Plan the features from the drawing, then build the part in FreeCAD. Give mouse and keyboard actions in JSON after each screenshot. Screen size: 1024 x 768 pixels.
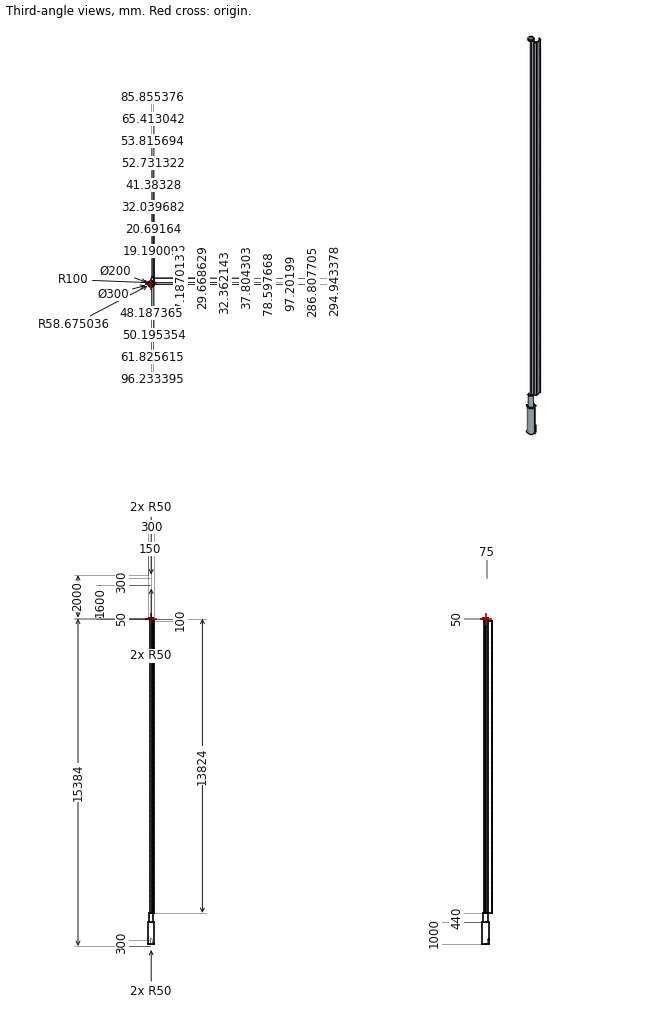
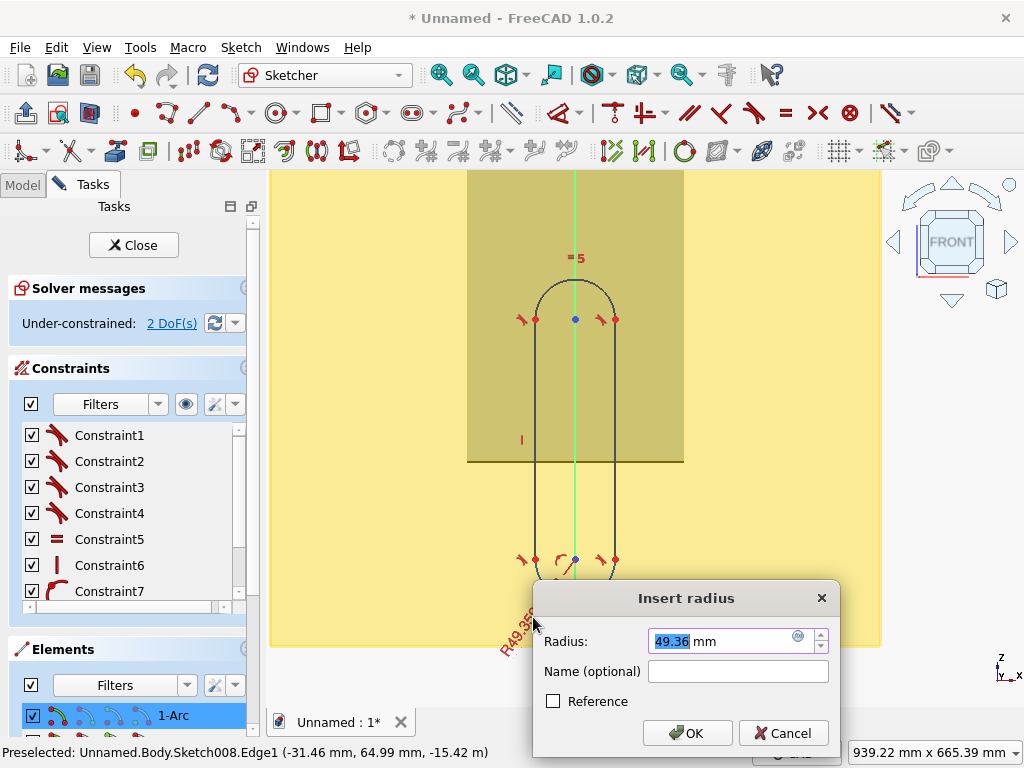
{"action": "type", "text": "50"}
{"action": "key", "text": "Return"}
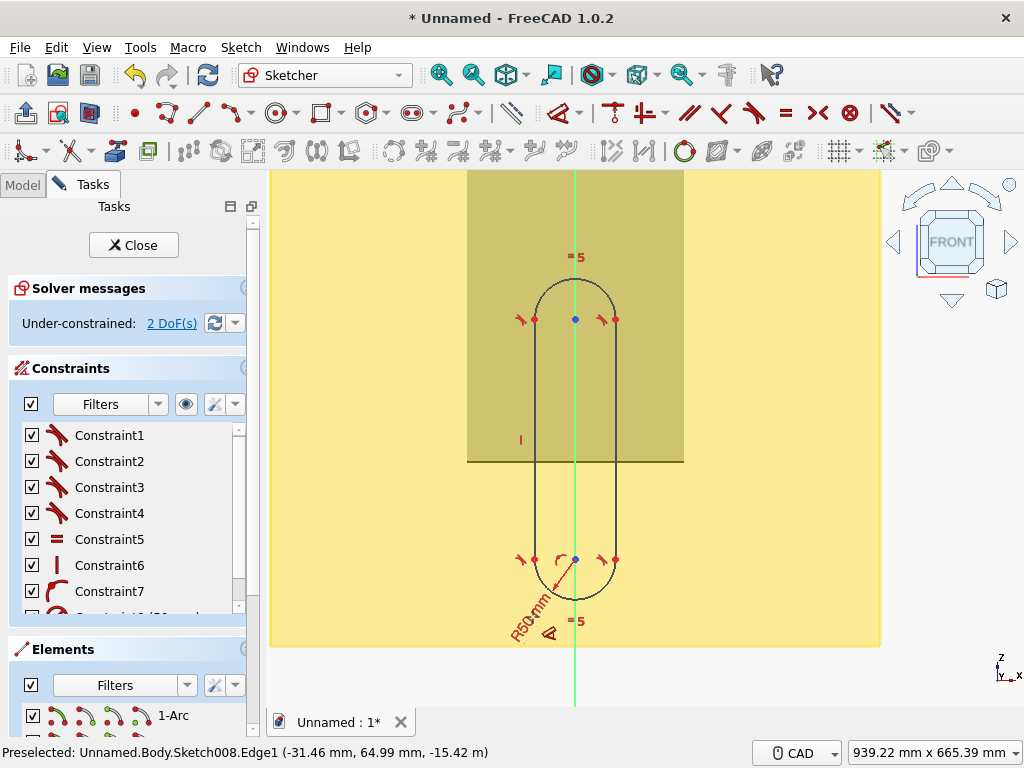
{"action": "left_click", "coordinate": [535, 487]}
{"action": "left_click", "coordinate": [501, 439]}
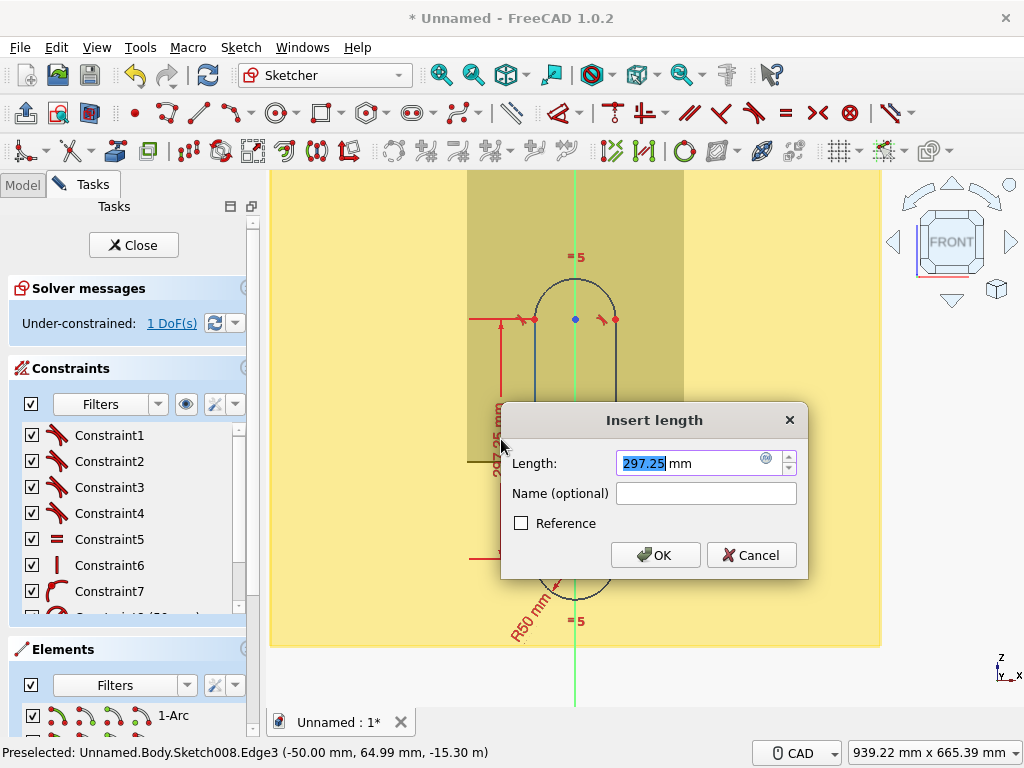
{"action": "type", "text": "300"}
{"action": "key", "text": "Return"}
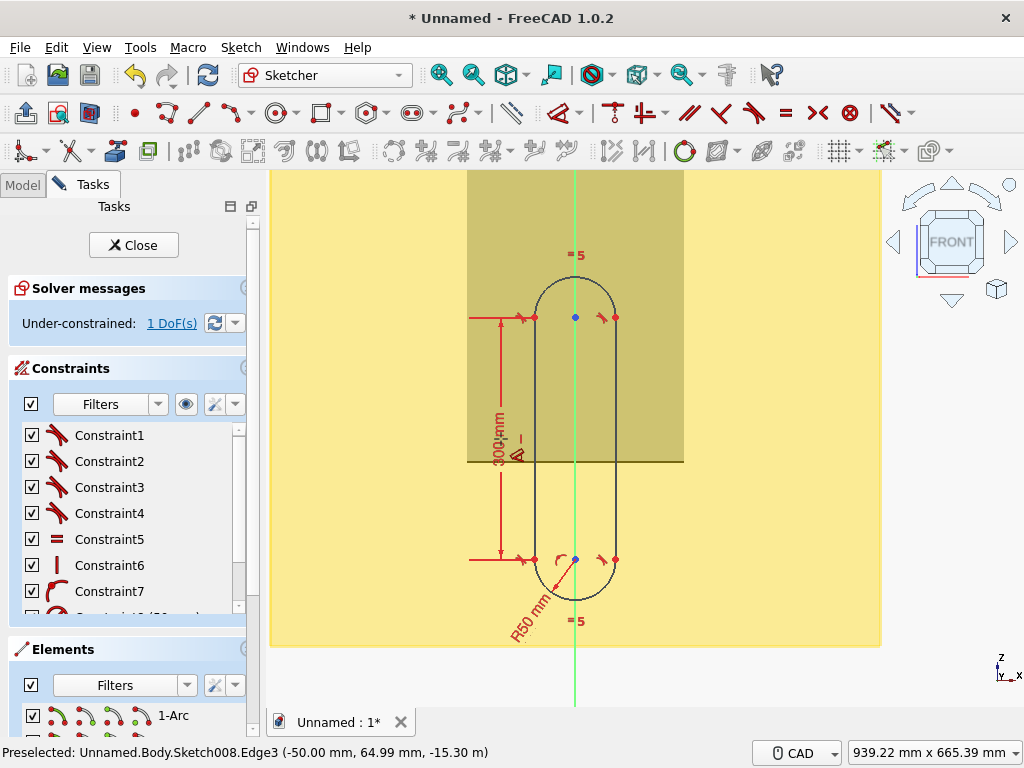
{"action": "left_click", "coordinate": [535, 560]}
{"action": "left_click", "coordinate": [501, 379]}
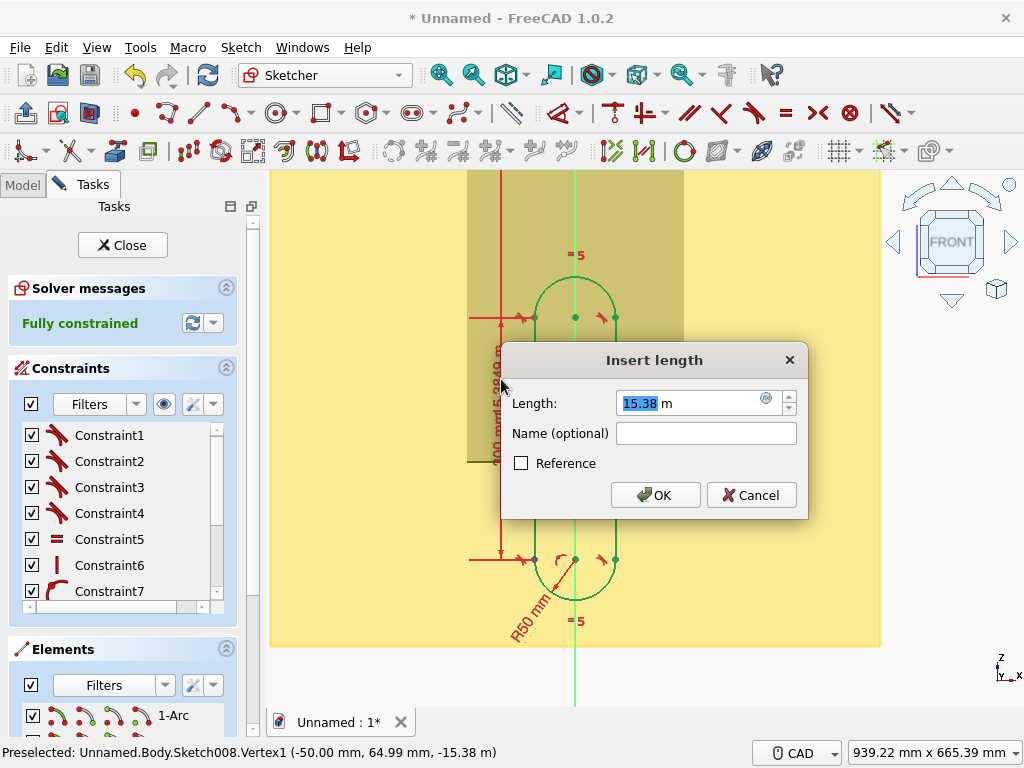
{"action": "key", "text": "ctrl+a"}
{"action": "type", "text": "15384 mm"}
{"action": "key", "text": "Return"}
{"action": "key", "text": "Escape"}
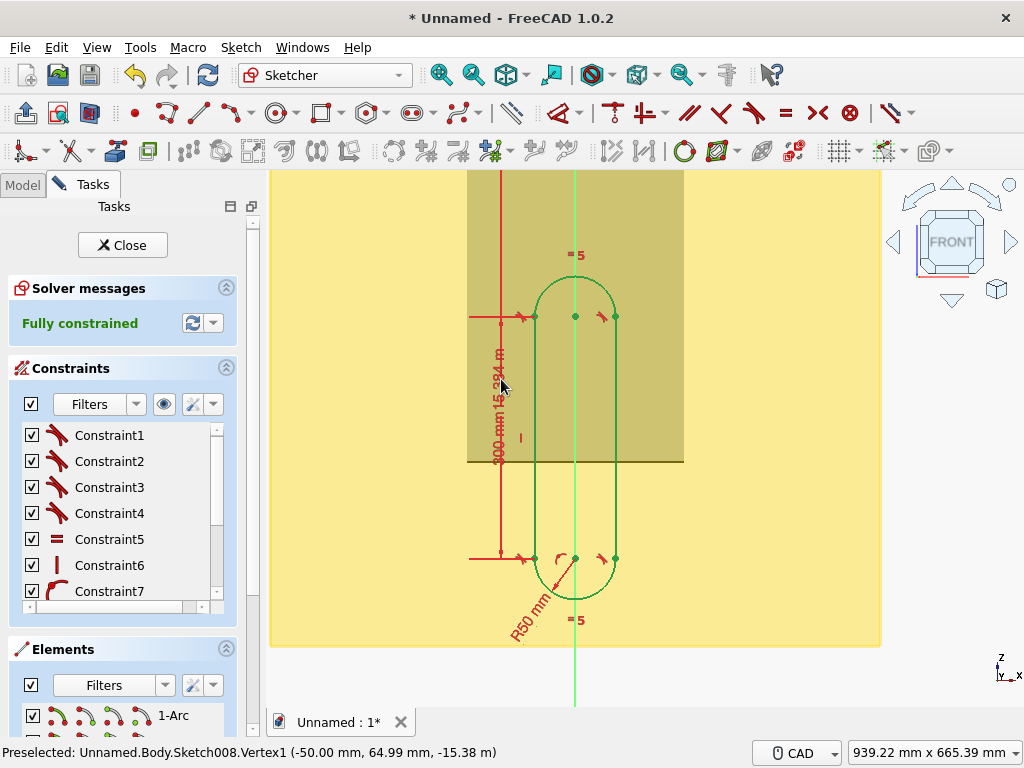
{"action": "left_click", "coordinate": [123, 245]}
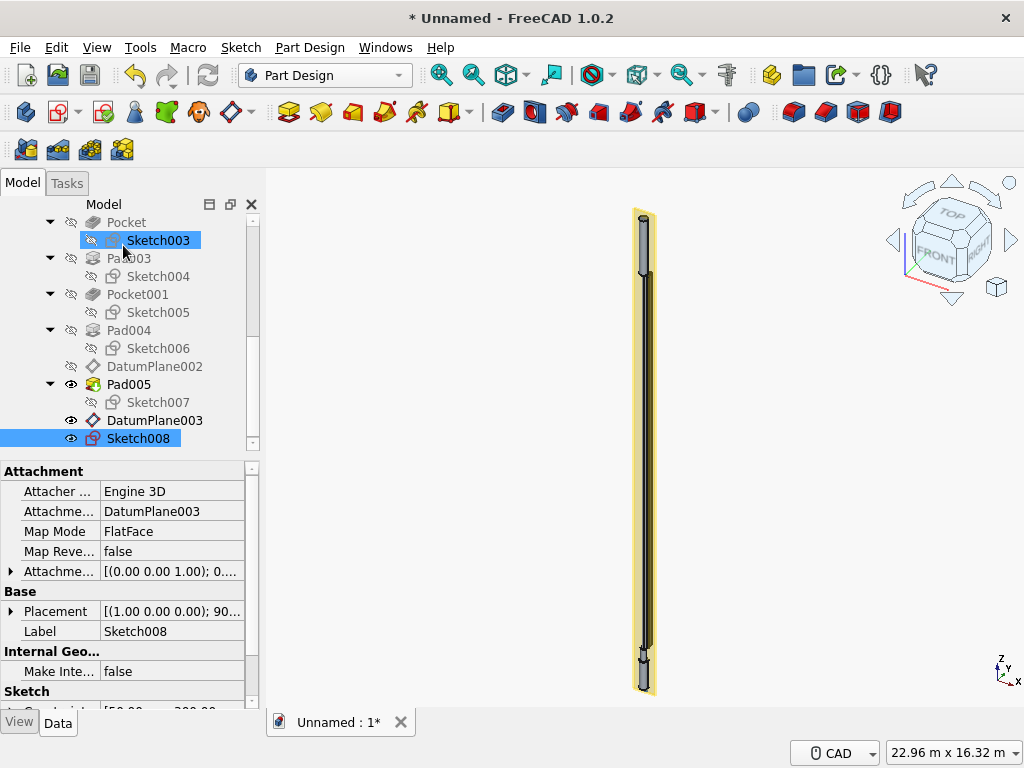
{"action": "left_click", "coordinate": [504, 112]}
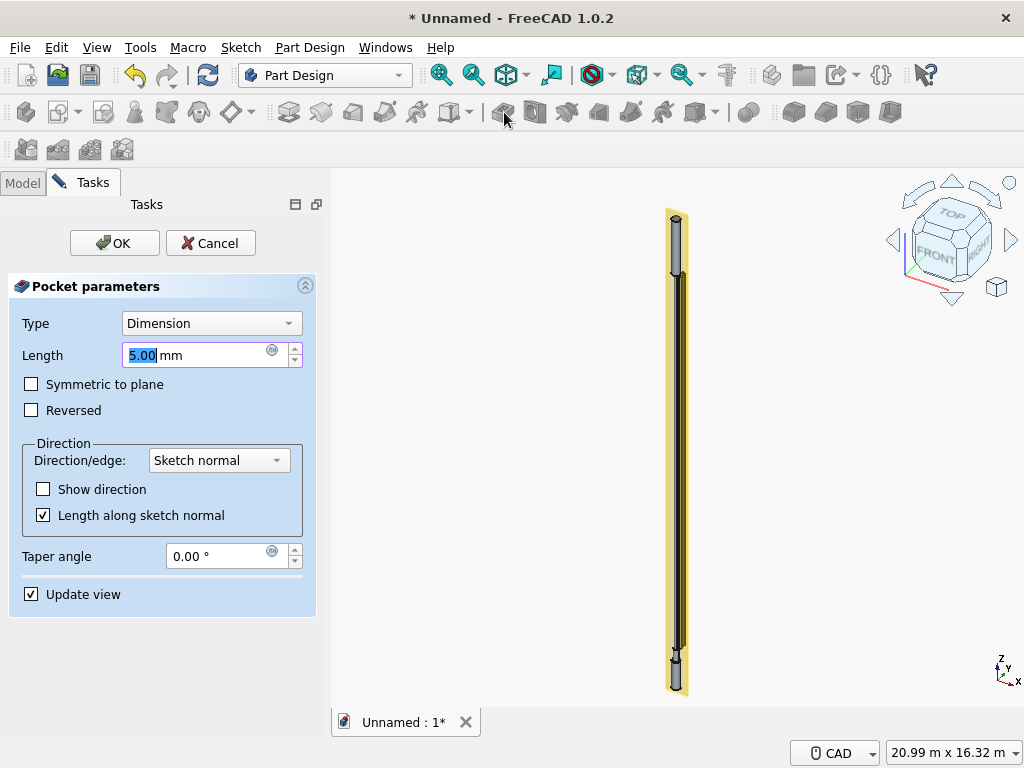
{"action": "type", "text": "300"}
{"action": "key", "text": "Tab"}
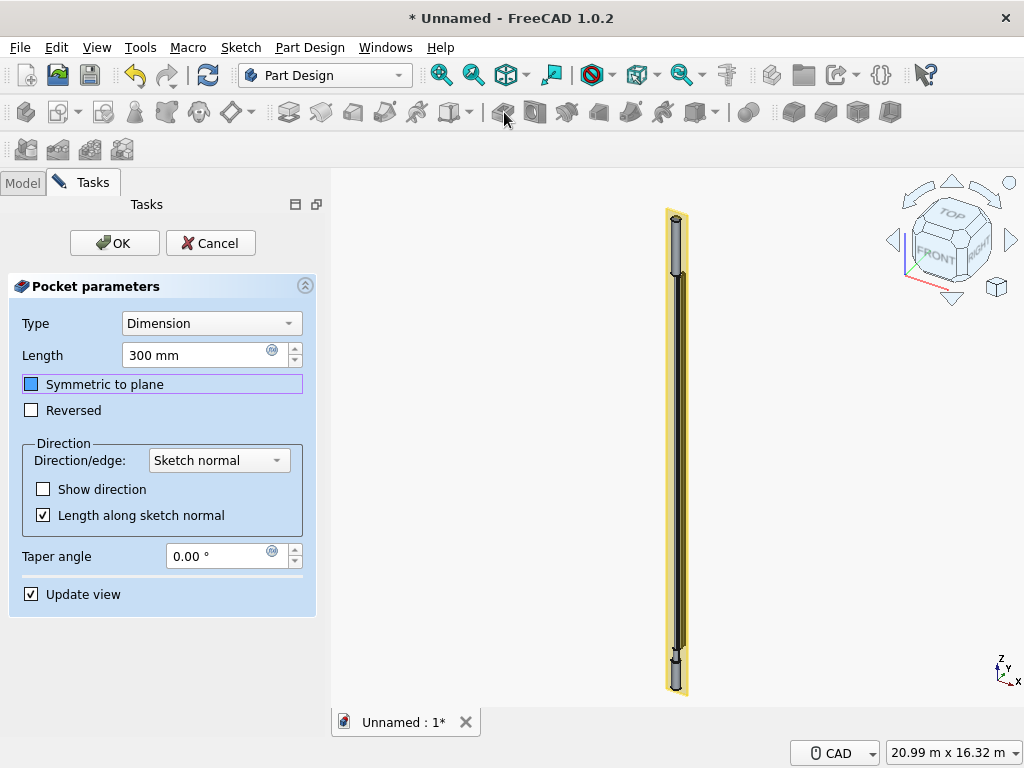
{"action": "left_click", "coordinate": [115, 243]}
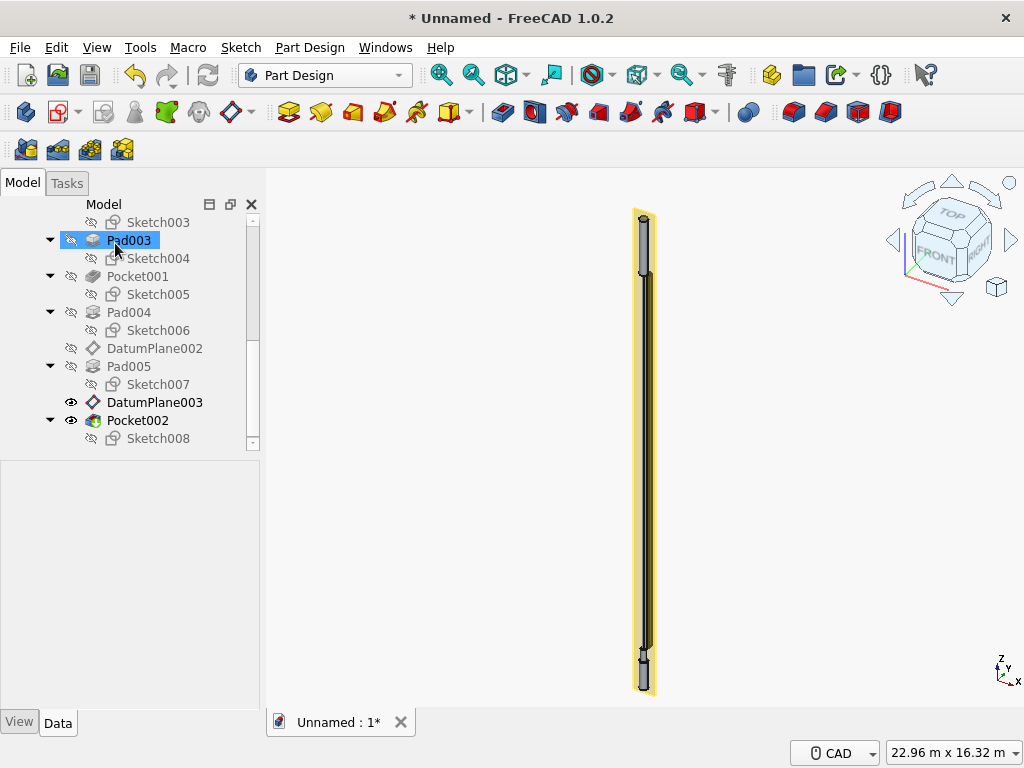
{"action": "left_click", "coordinate": [116, 402]}
{"action": "key", "text": "space"}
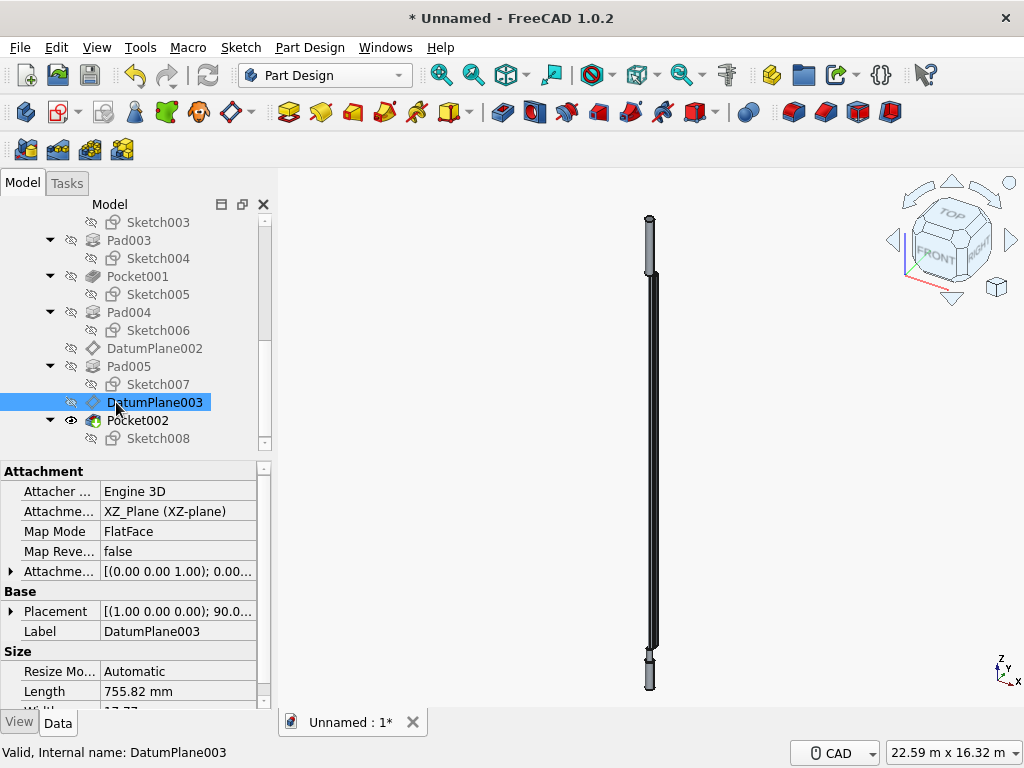
{"action": "left_click", "coordinate": [318, 667]}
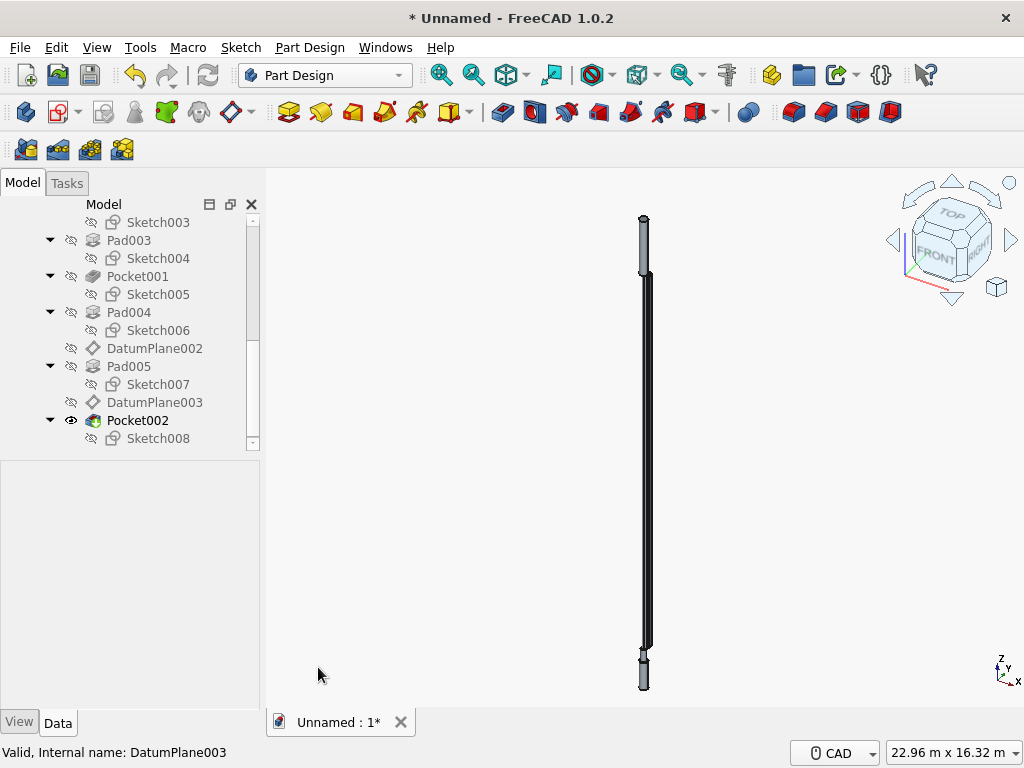
{"action": "left_click", "coordinate": [58, 112]}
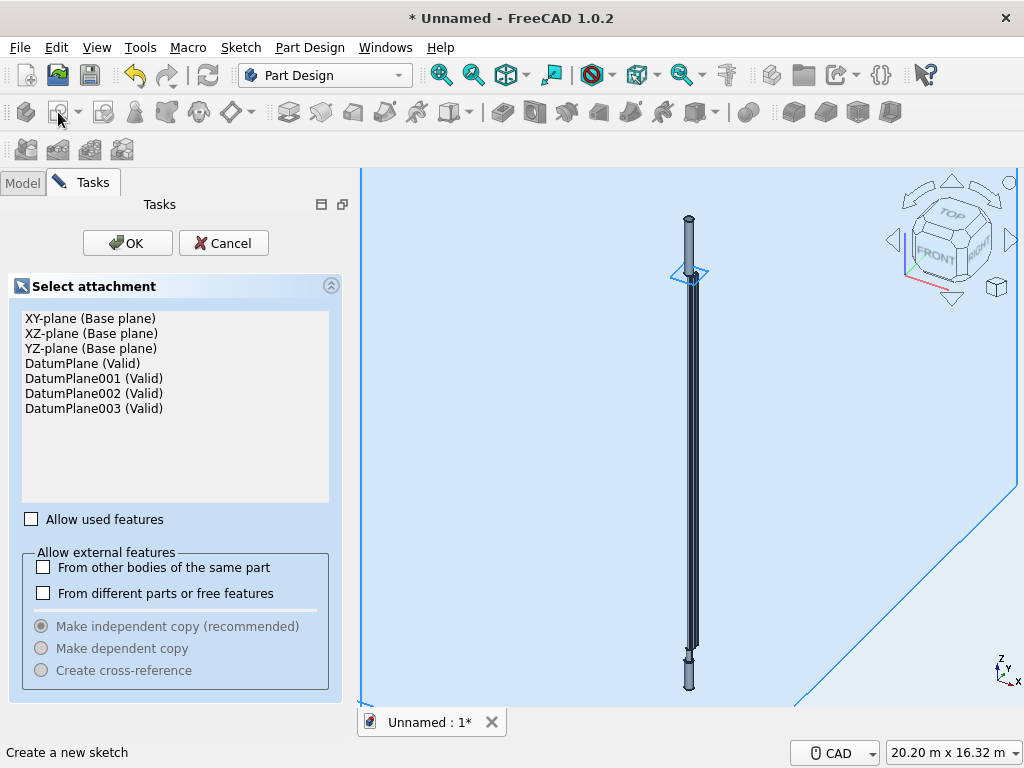
{"action": "left_click", "coordinate": [82, 334]}